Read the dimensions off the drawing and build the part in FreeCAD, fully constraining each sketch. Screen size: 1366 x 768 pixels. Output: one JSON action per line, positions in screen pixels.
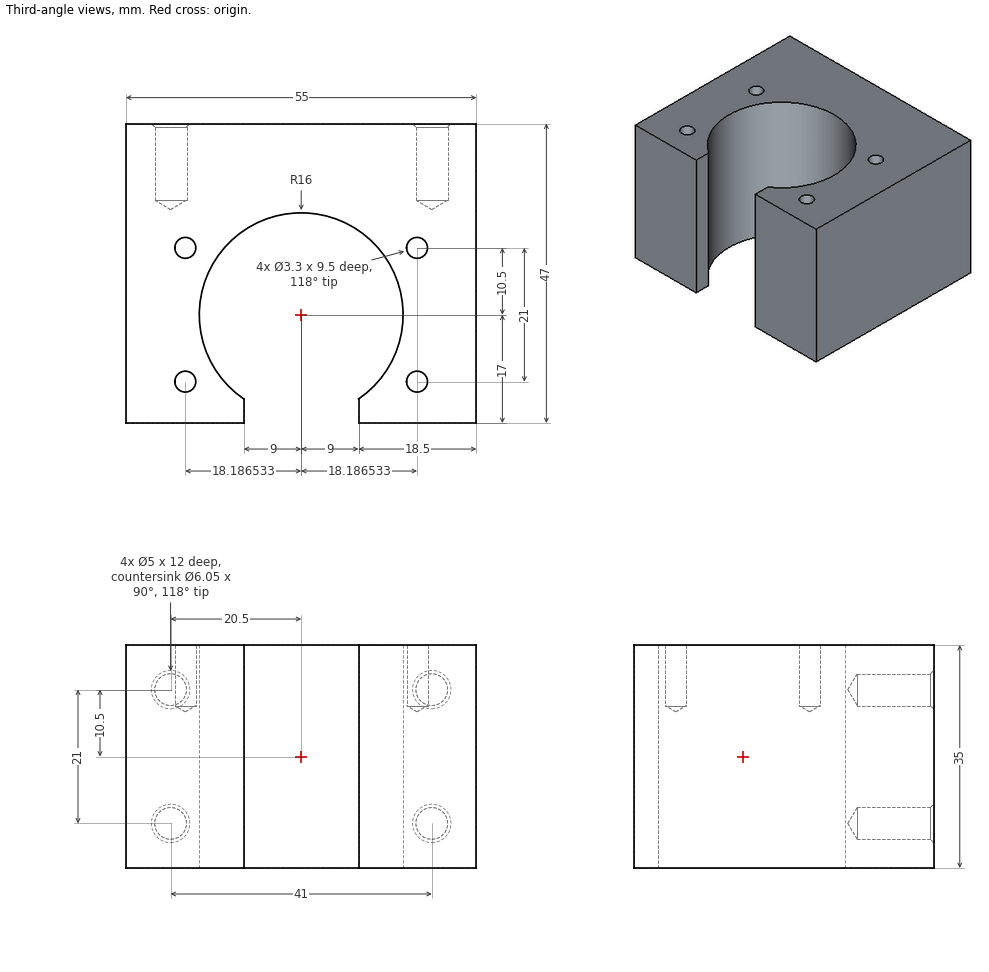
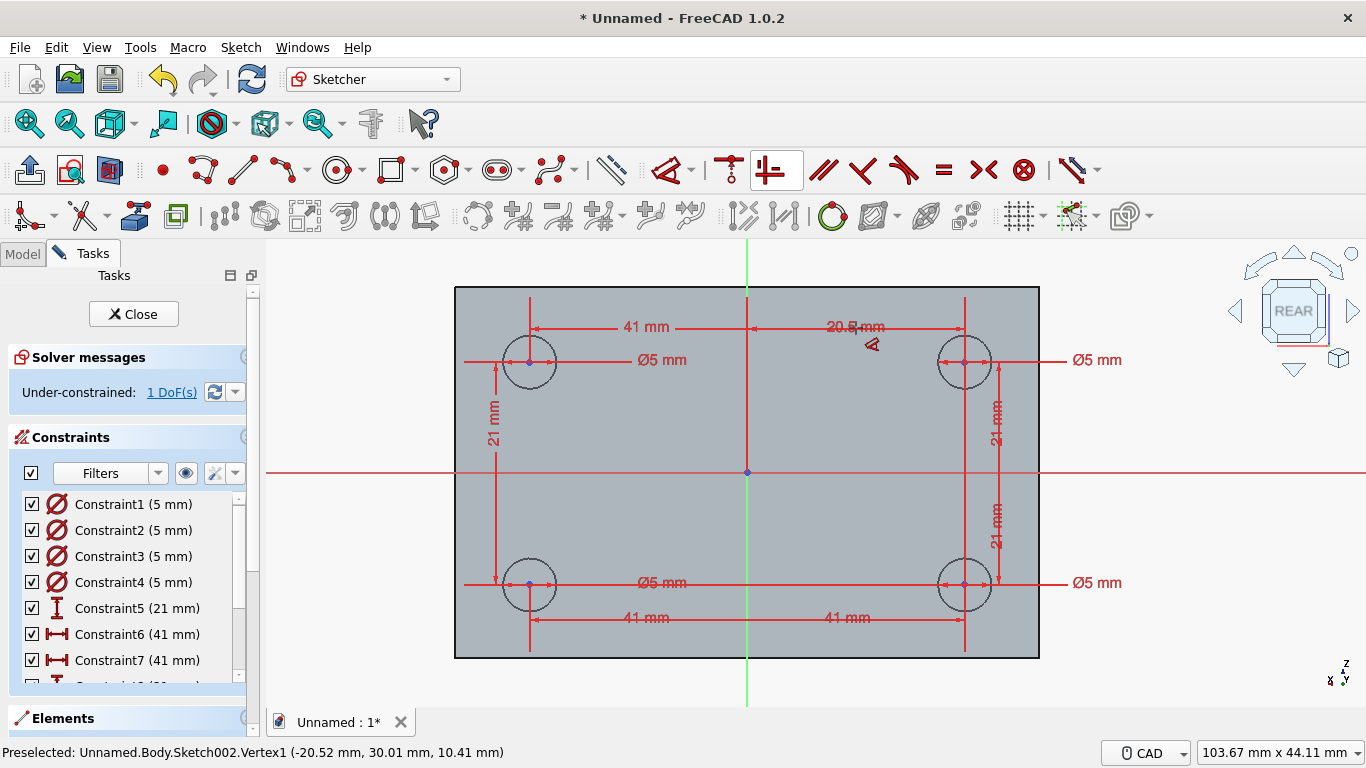
{"action": "left_click", "coordinate": [965, 362]}
{"action": "left_click", "coordinate": [999, 392]}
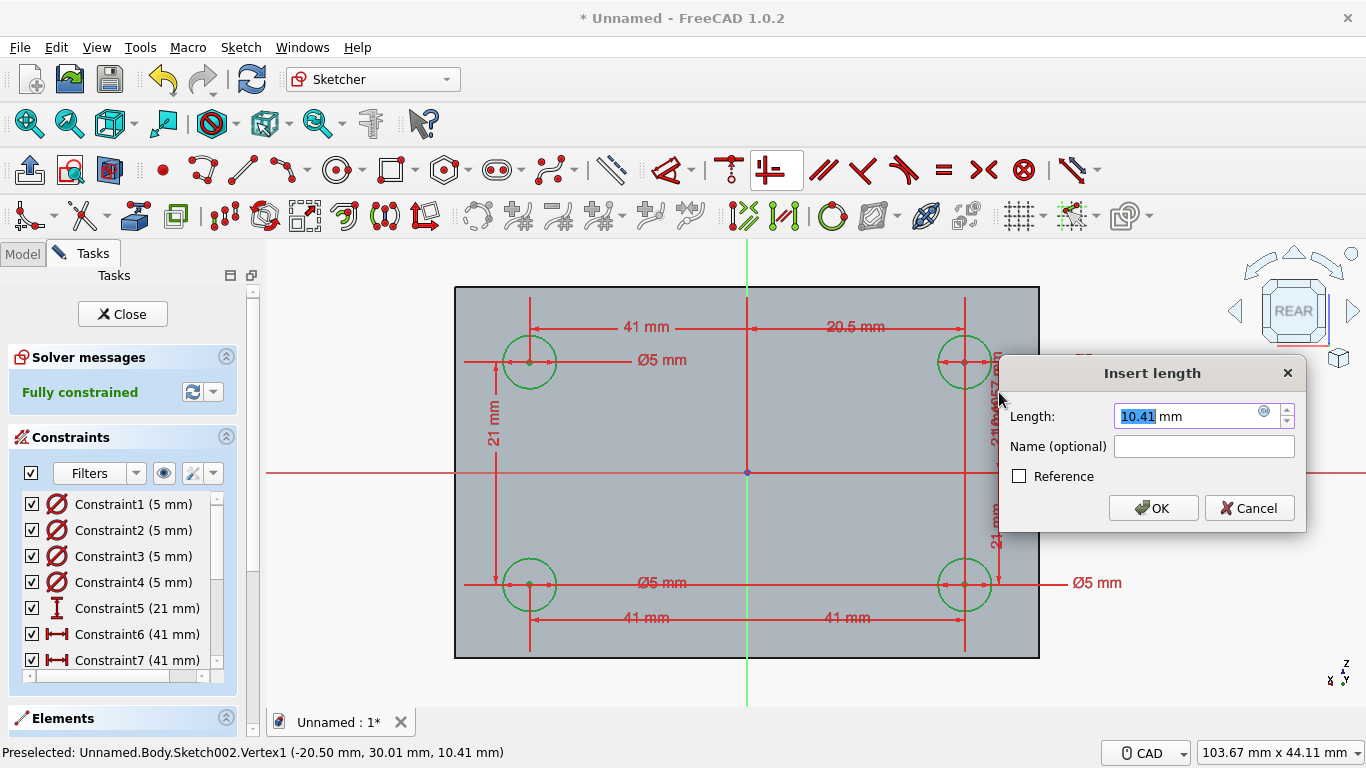
{"action": "type", "text": "10.5"}
{"action": "key", "text": "Return"}
{"action": "key", "text": "Escape"}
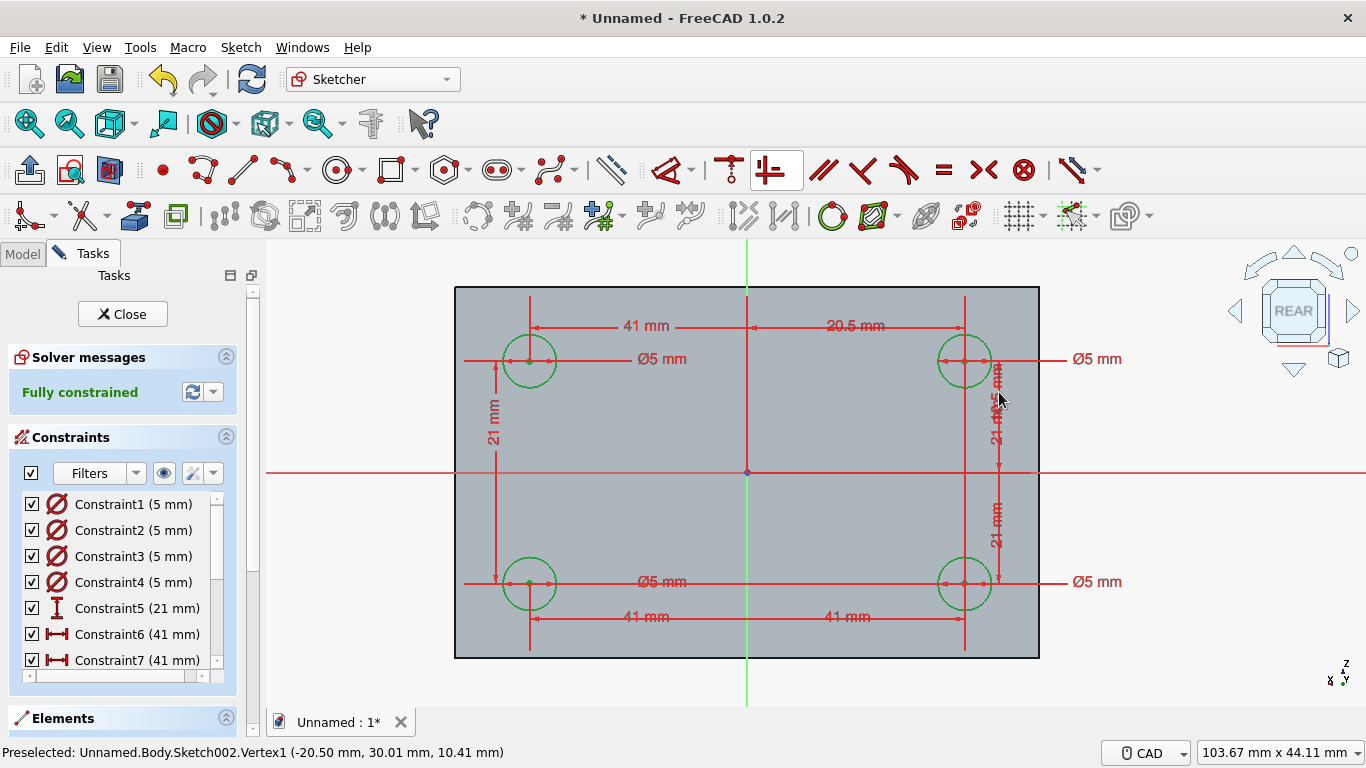
{"action": "left_click", "coordinate": [123, 314]}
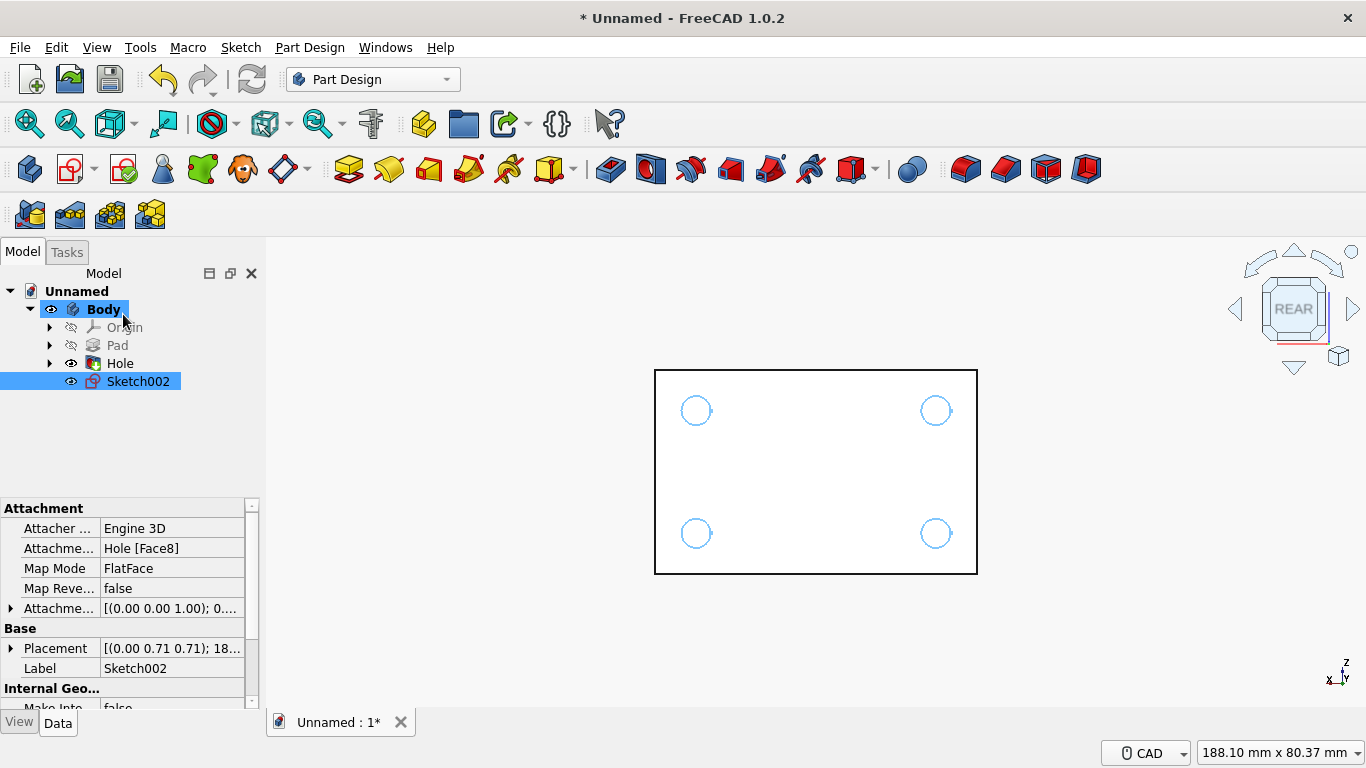
{"action": "left_click", "coordinate": [652, 170]}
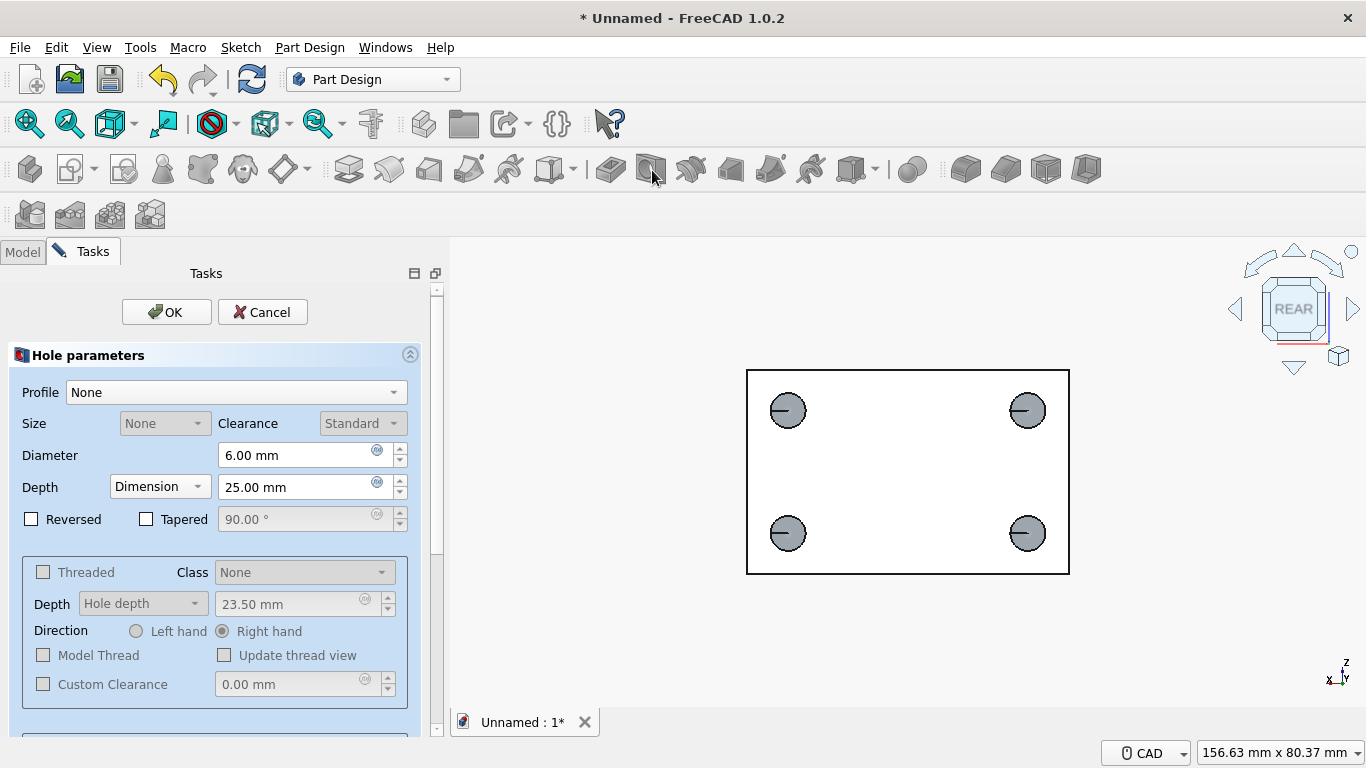
{"action": "triple_click", "coordinate": [305, 455]}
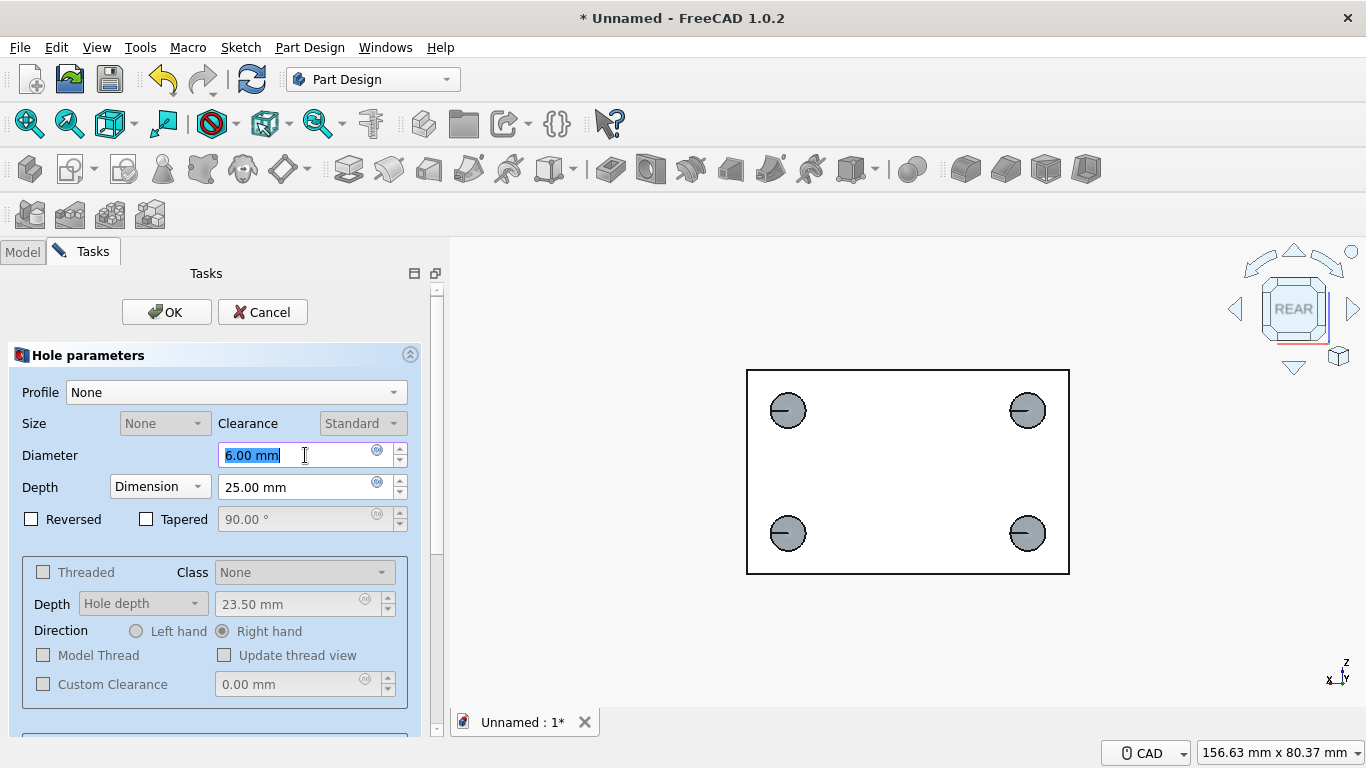
{"action": "type", "text": "5"}
{"action": "key", "text": "Tab"}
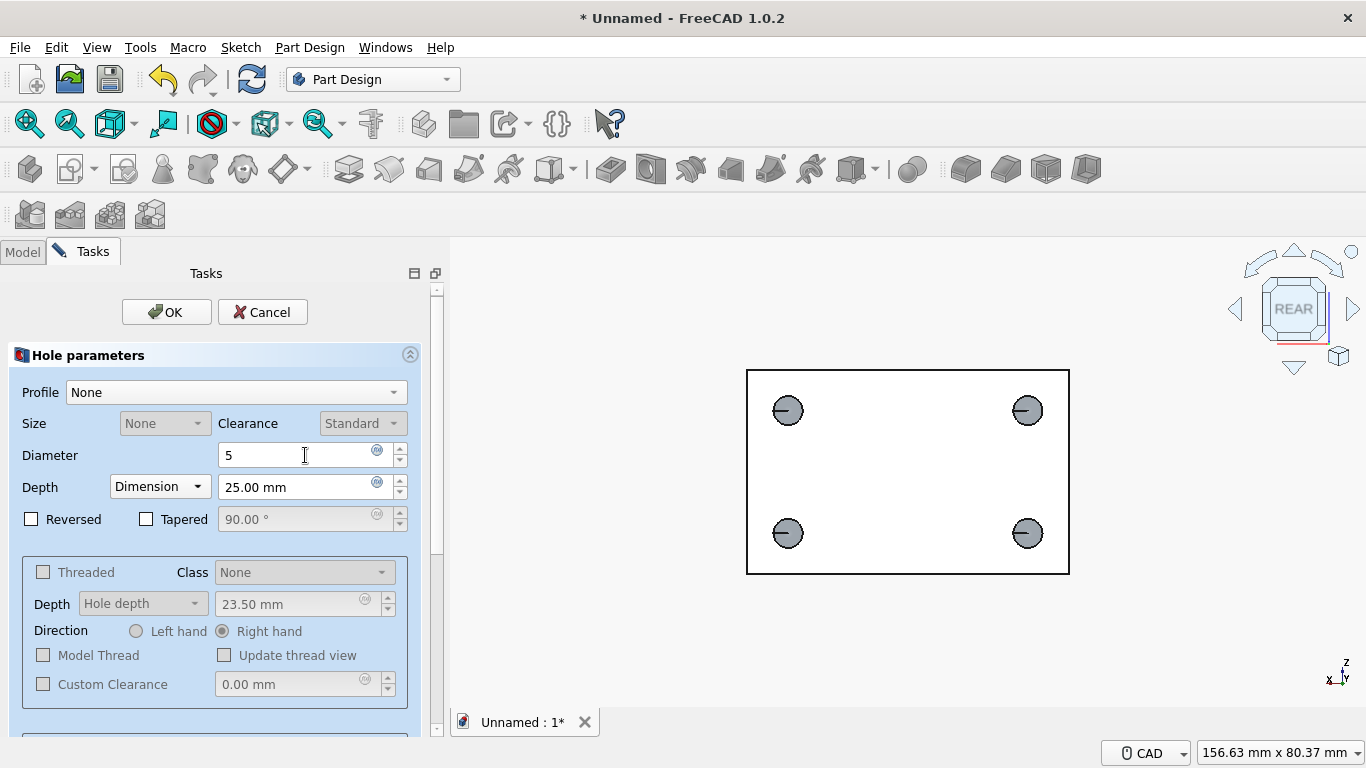
{"action": "triple_click", "coordinate": [305, 487]}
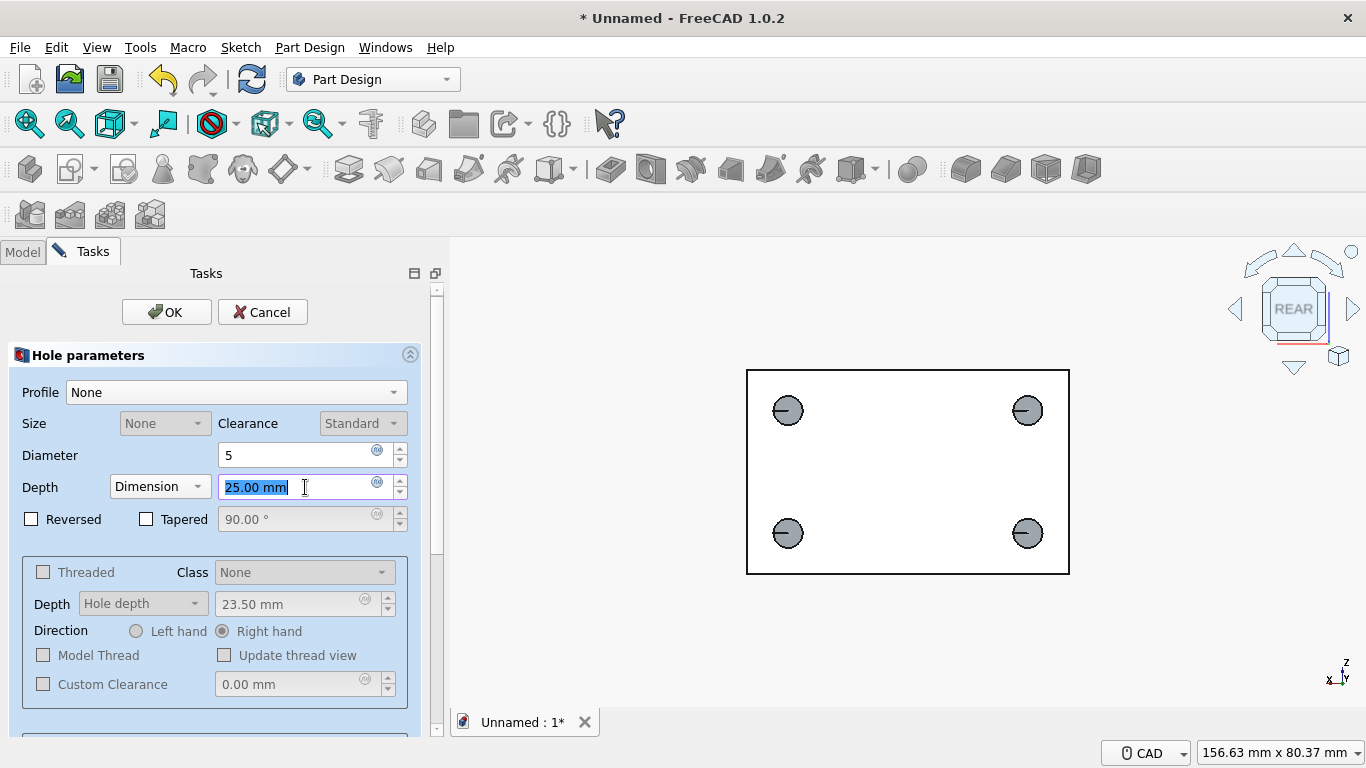
{"action": "type", "text": "12"}
{"action": "key", "text": "Tab"}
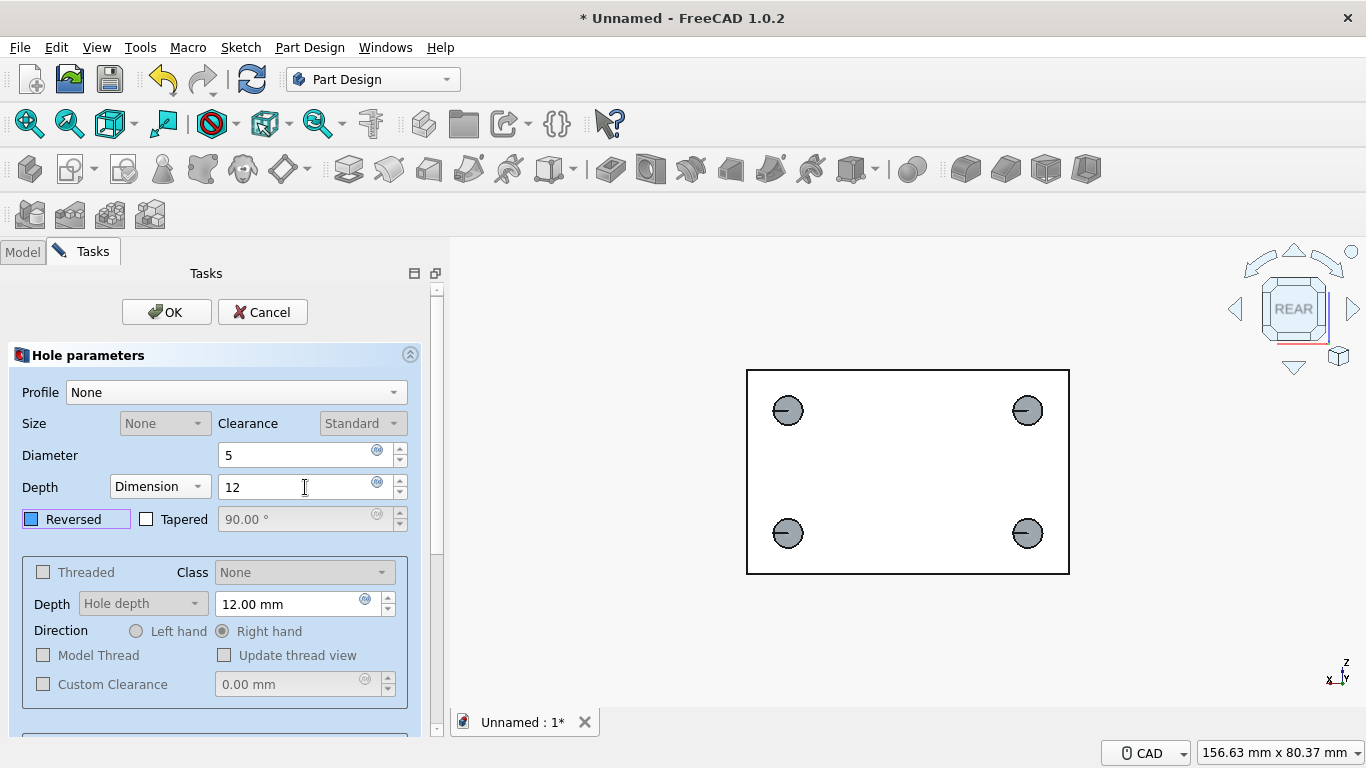
{"action": "scroll", "coordinate": [437, 510], "scroll_direction": "down", "scroll_amount": 2}